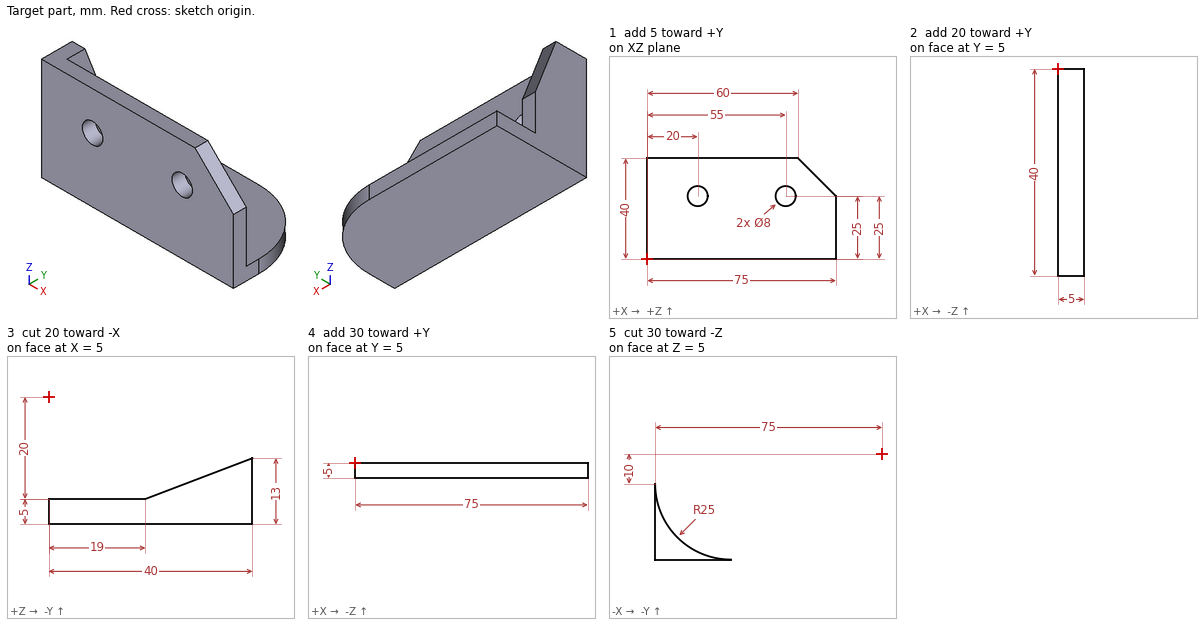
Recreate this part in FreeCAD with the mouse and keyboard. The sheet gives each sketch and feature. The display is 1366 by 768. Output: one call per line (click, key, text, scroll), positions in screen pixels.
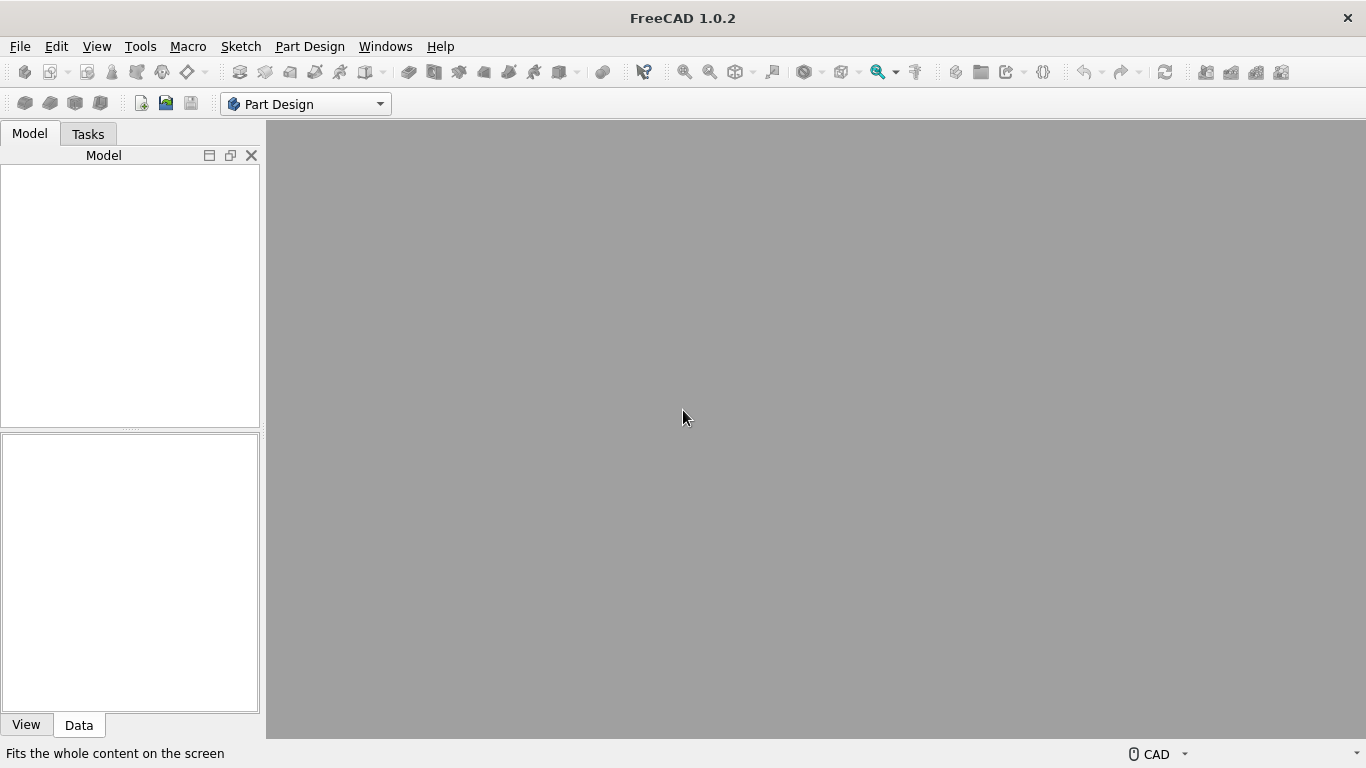
click(141, 104)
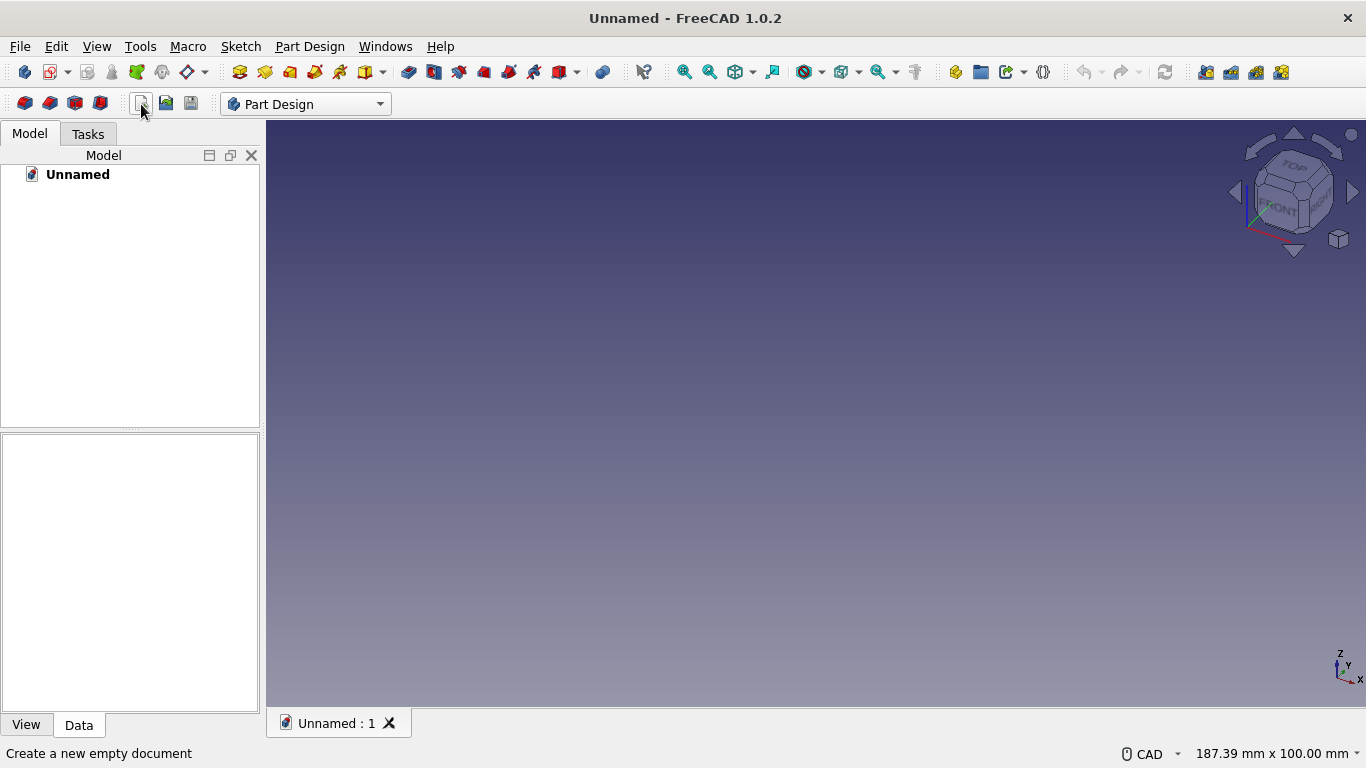
click(50, 72)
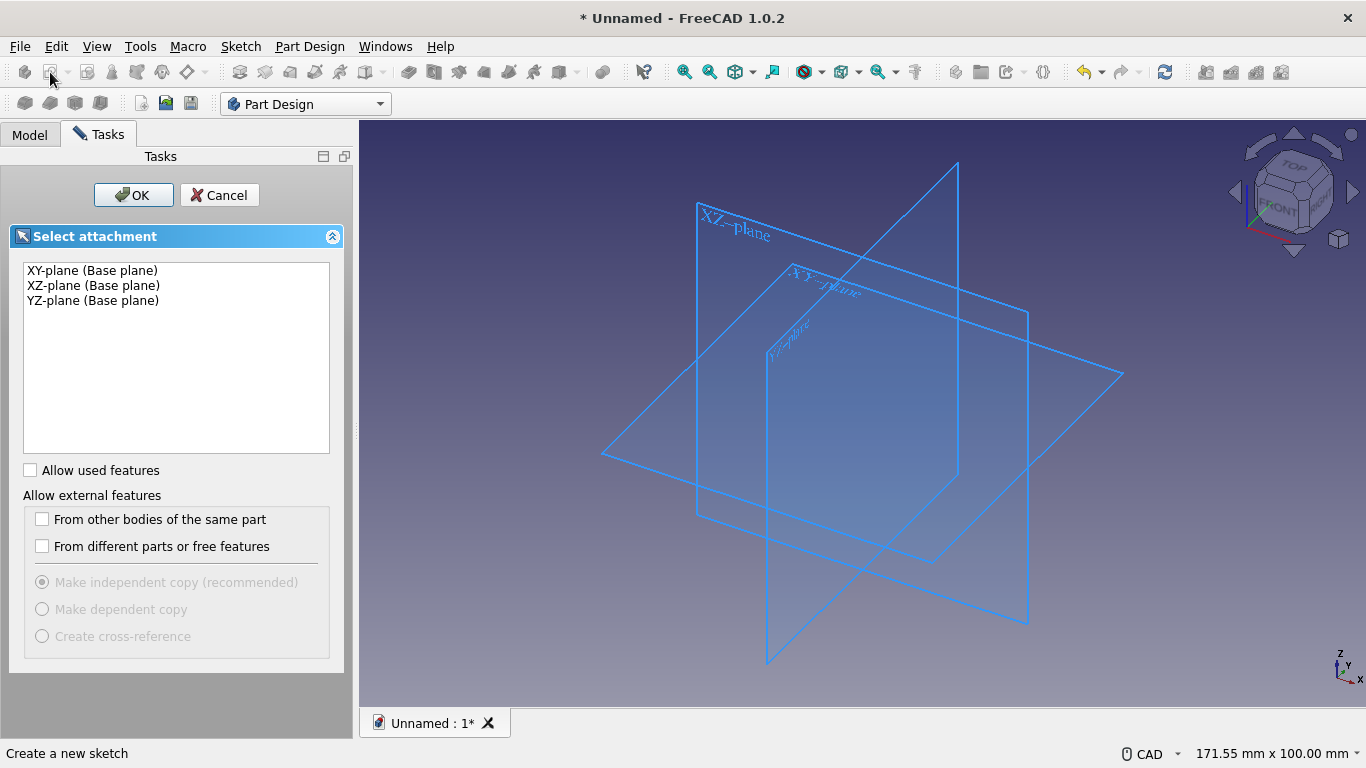
click(84, 286)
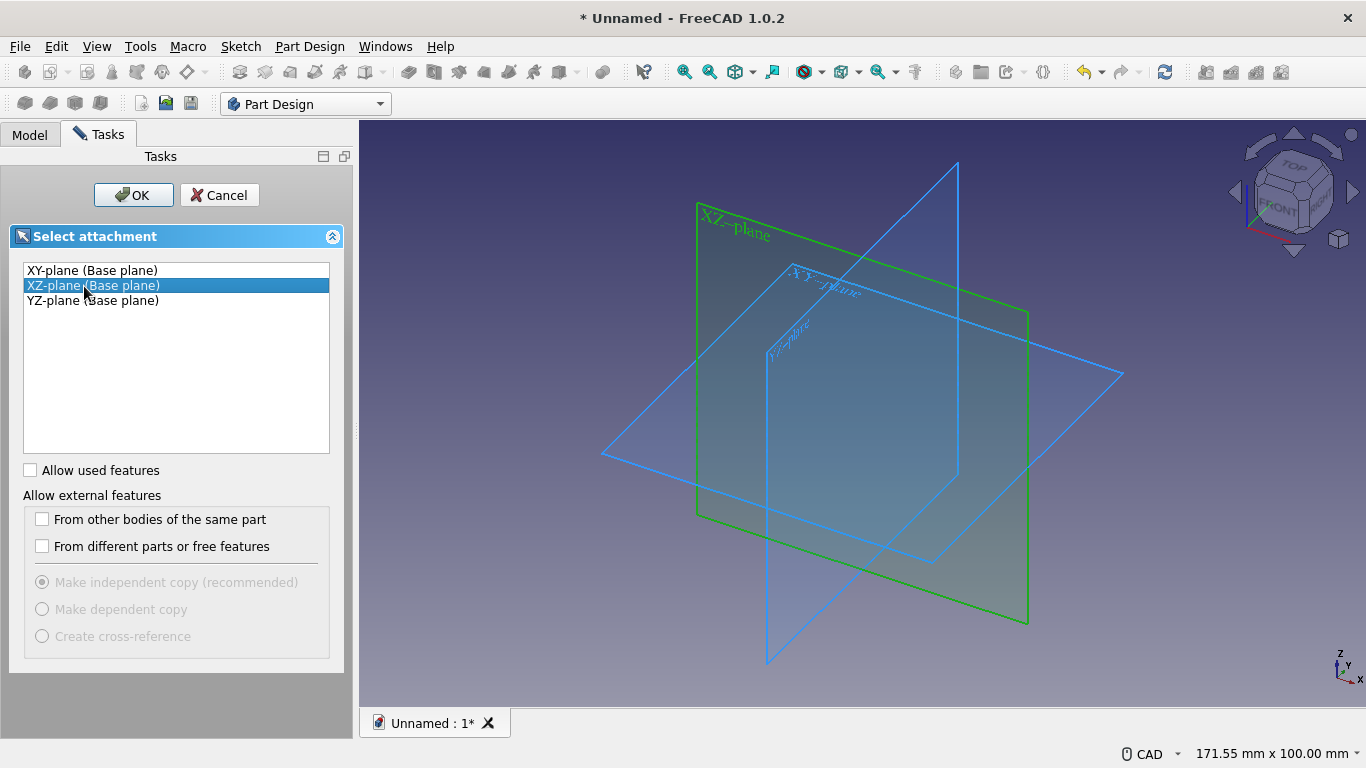
click(134, 195)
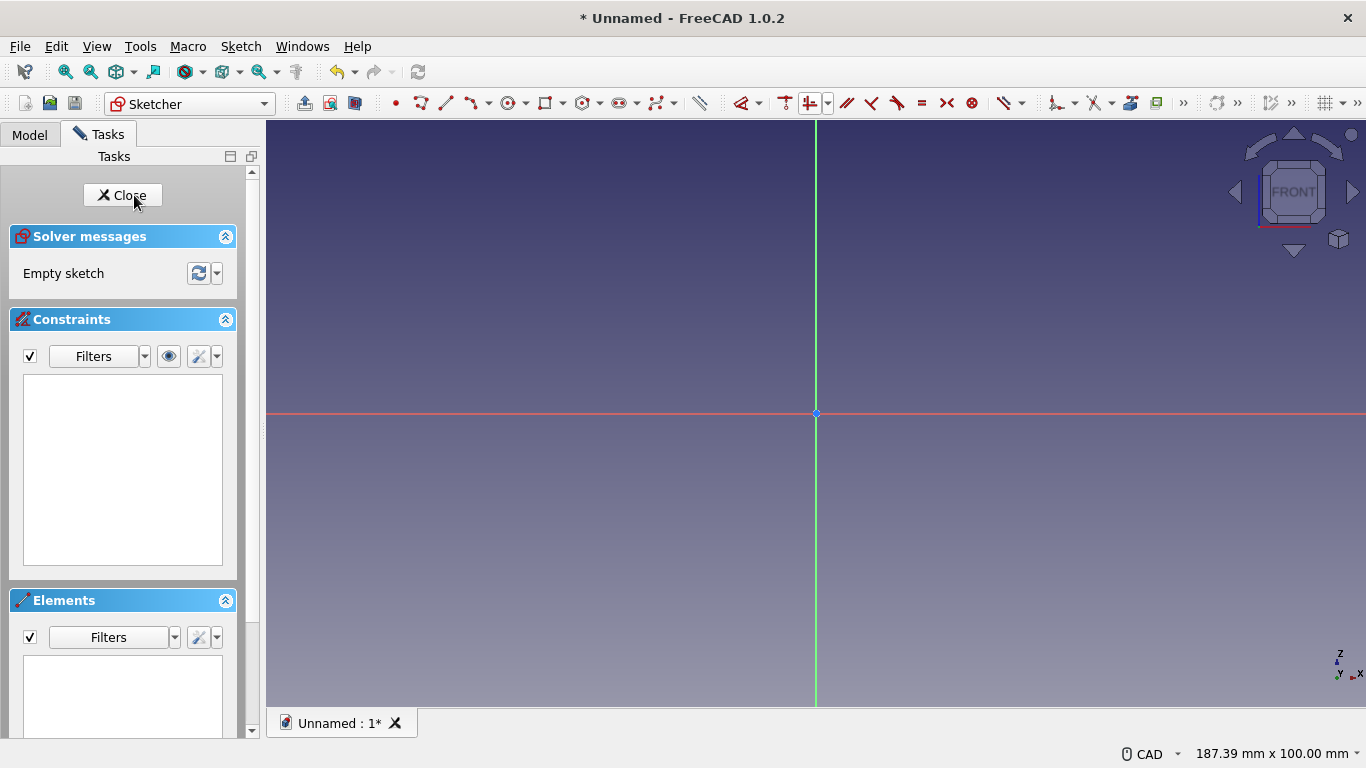
scroll(294, 679, down, 1)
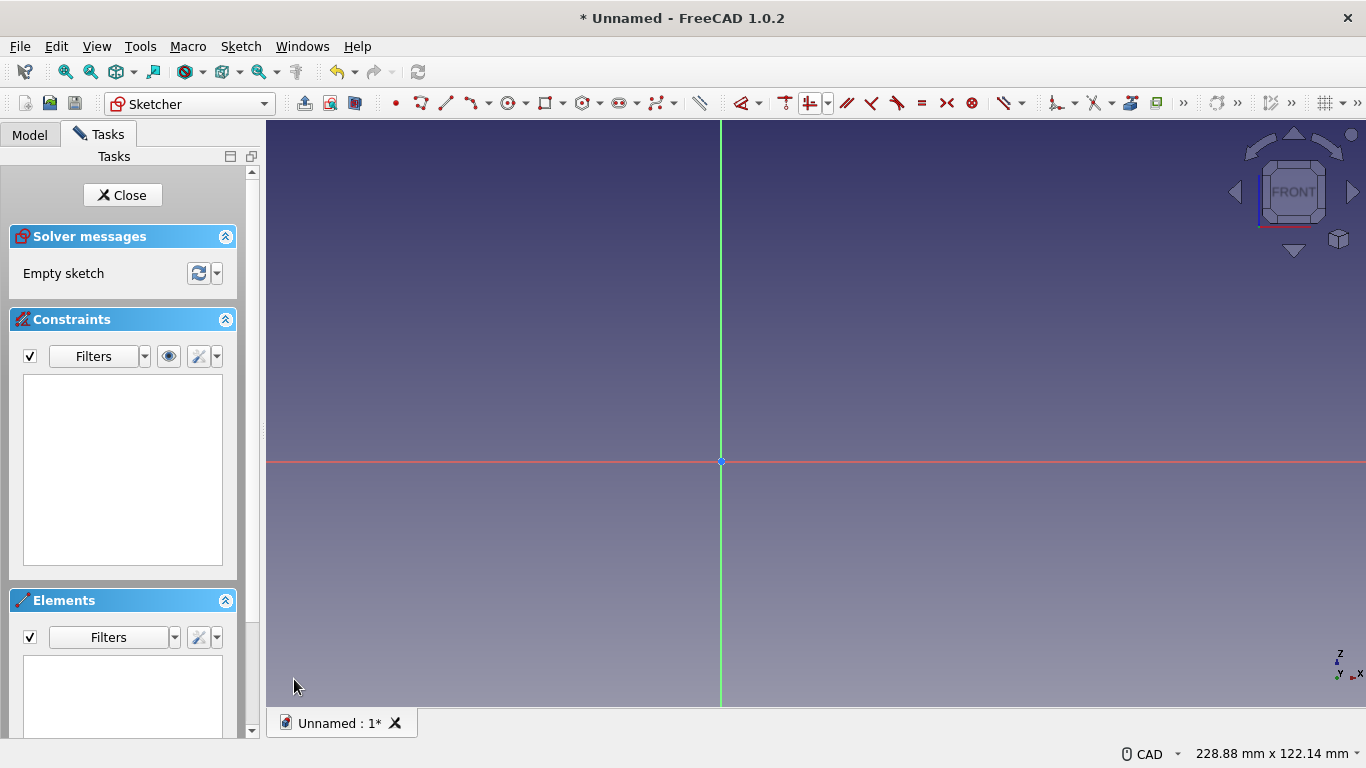
scroll(1089, 308, up, 3)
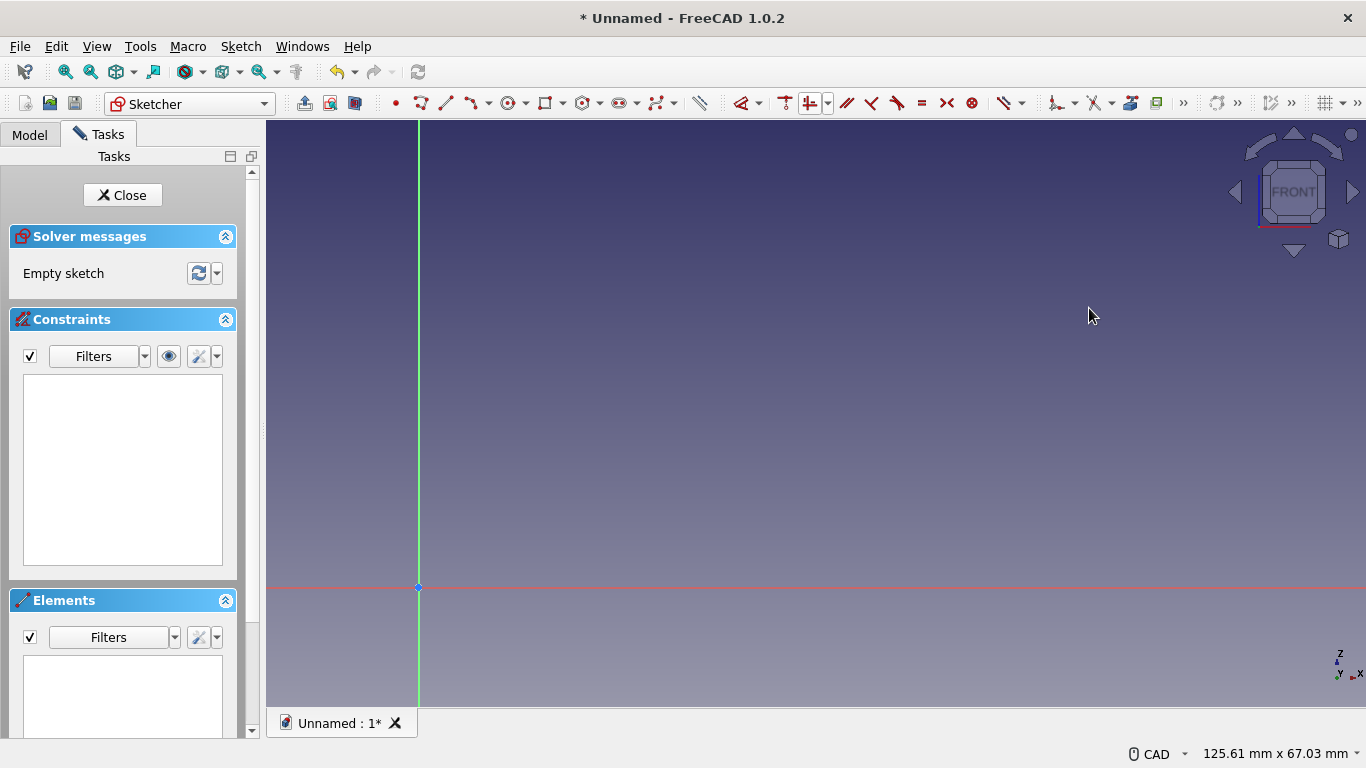
click(421, 104)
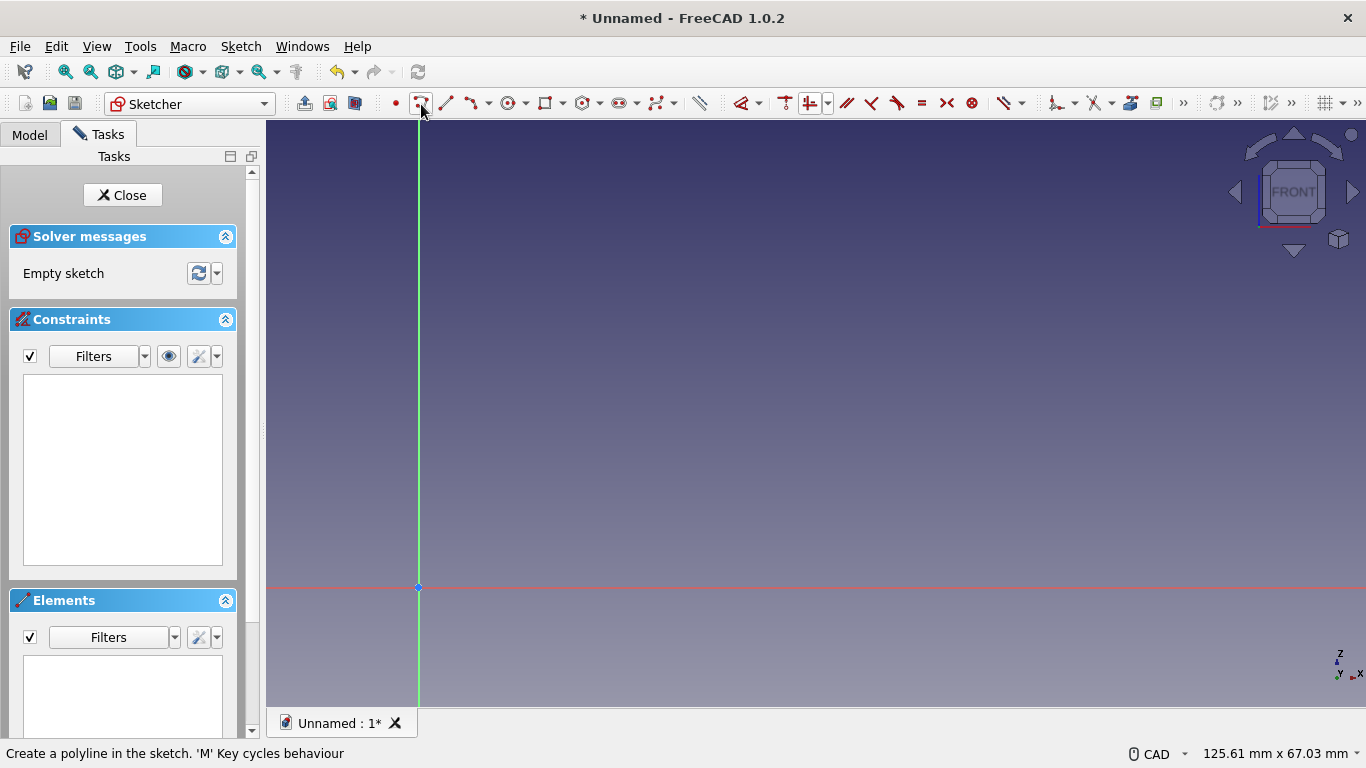
click(419, 588)
click(428, 238)
click(944, 238)
click(1075, 369)
click(1075, 579)
click(419, 588)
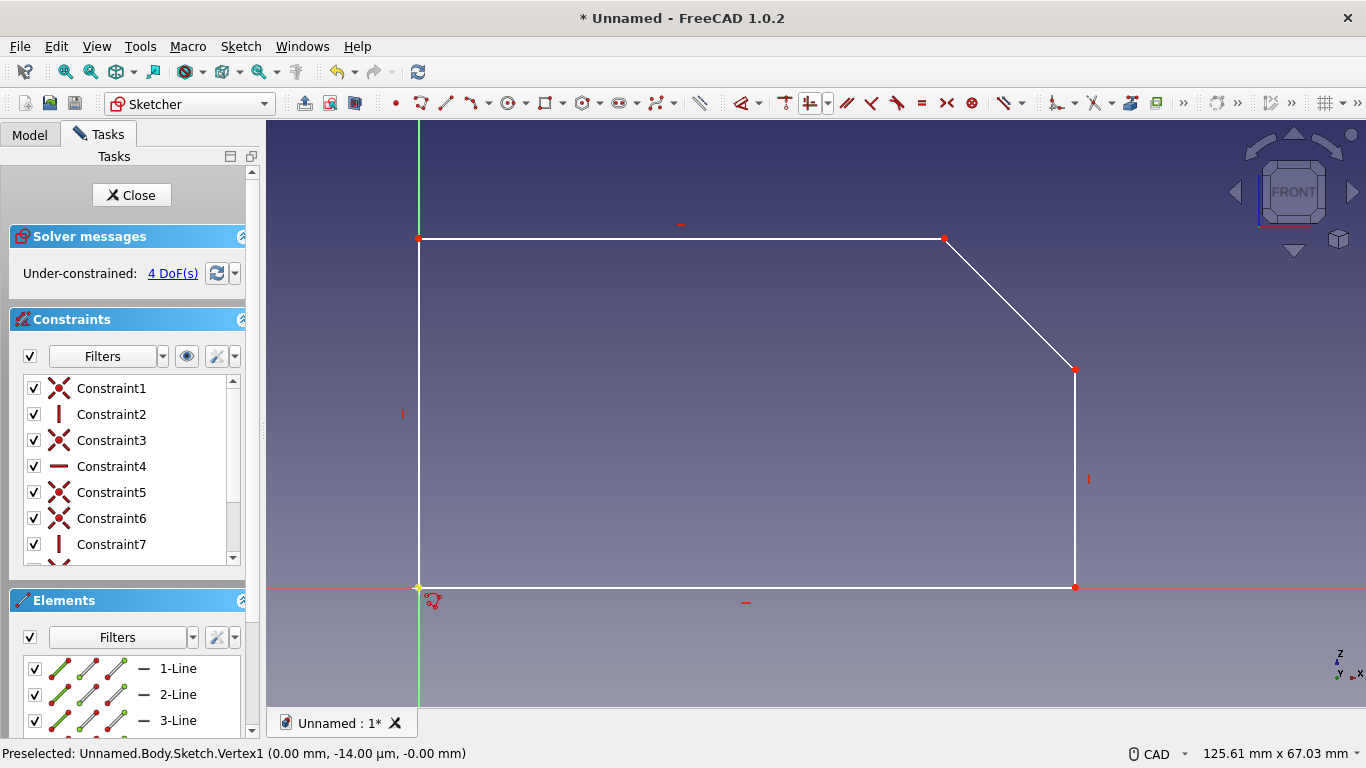
click(508, 104)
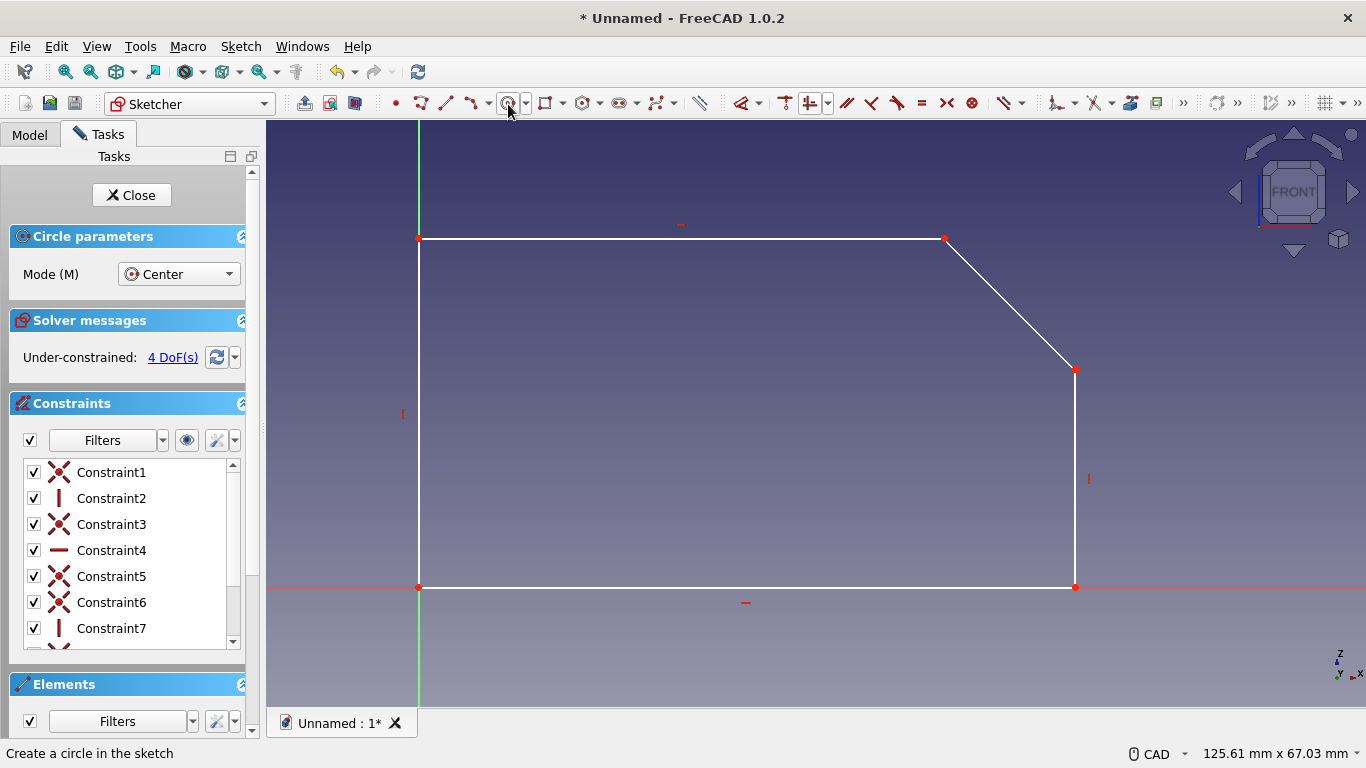
click(900, 369)
click(925, 344)